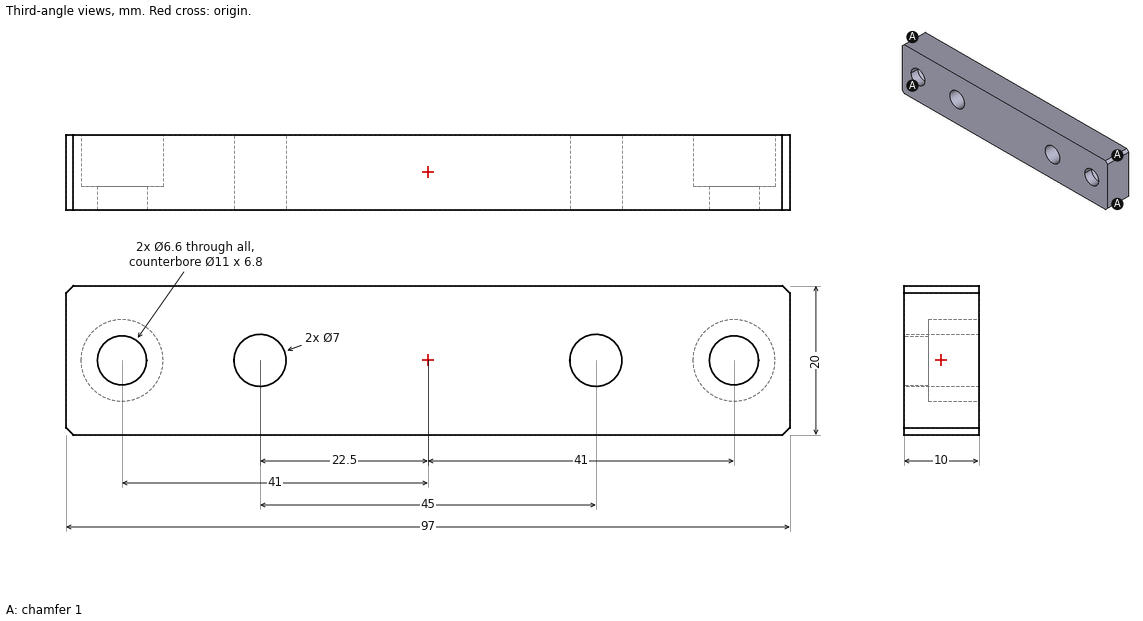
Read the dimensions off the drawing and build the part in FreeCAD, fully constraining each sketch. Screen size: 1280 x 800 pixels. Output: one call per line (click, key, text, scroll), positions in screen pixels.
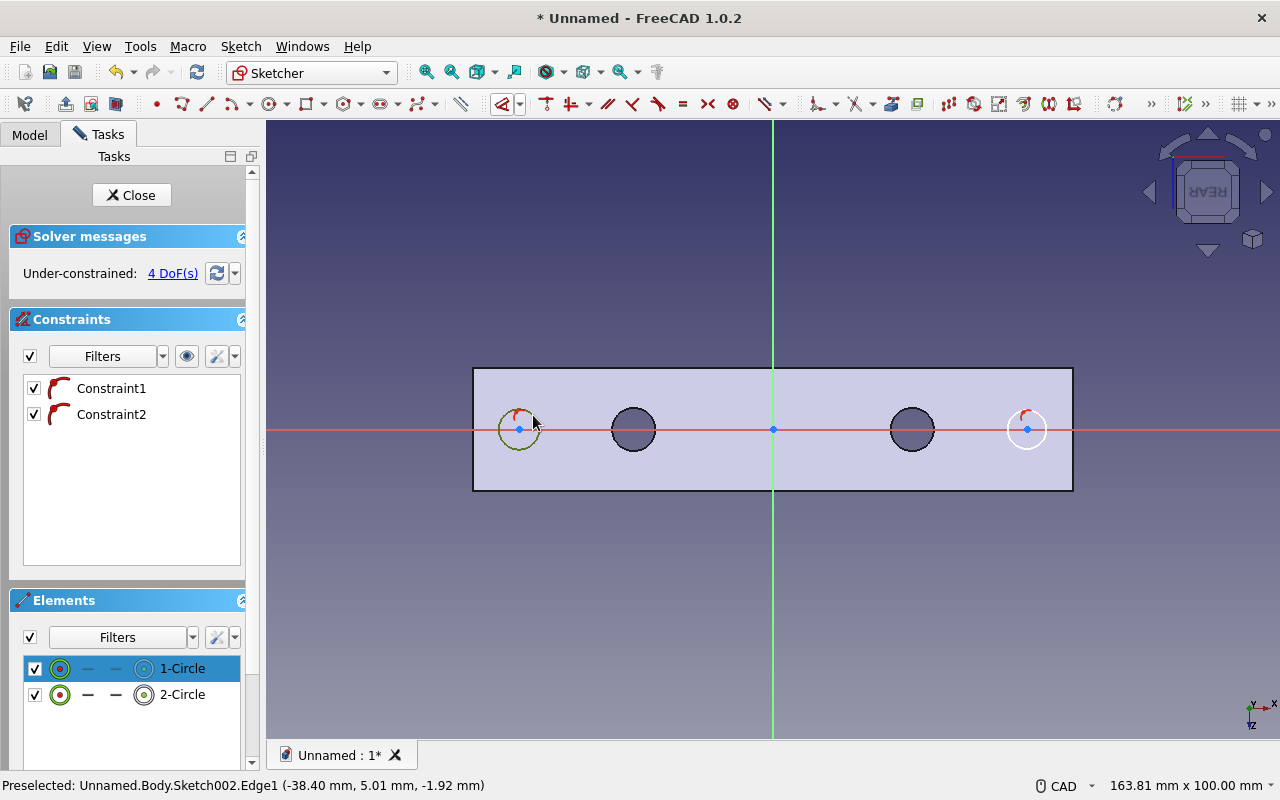
click(1041, 416)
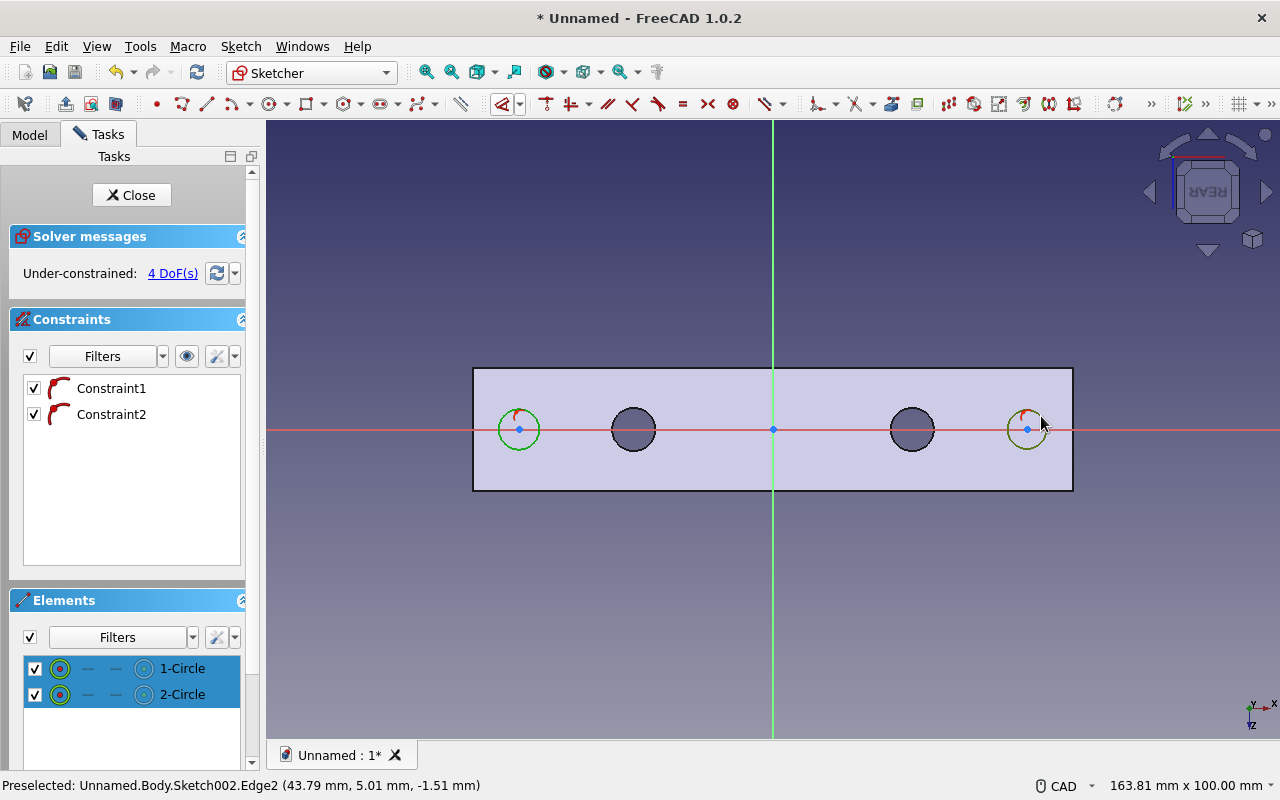
click(683, 104)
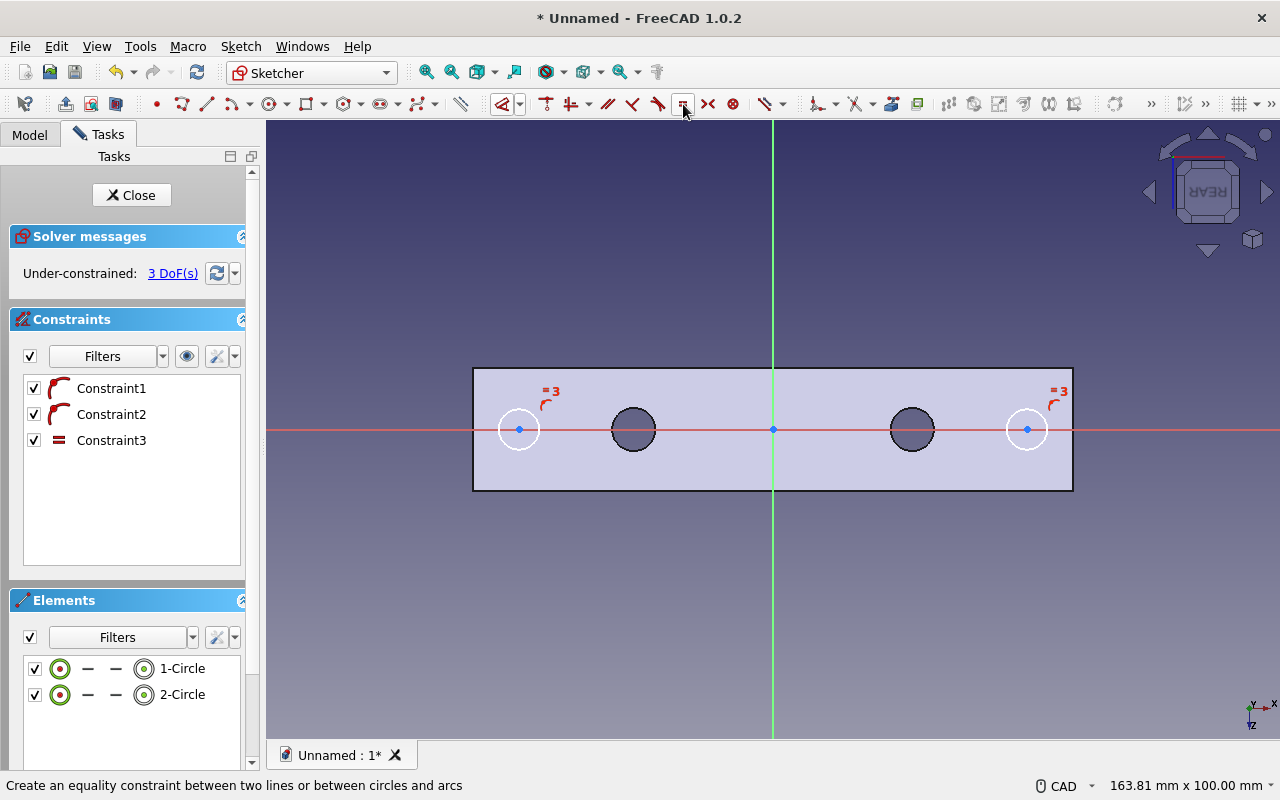
click(533, 415)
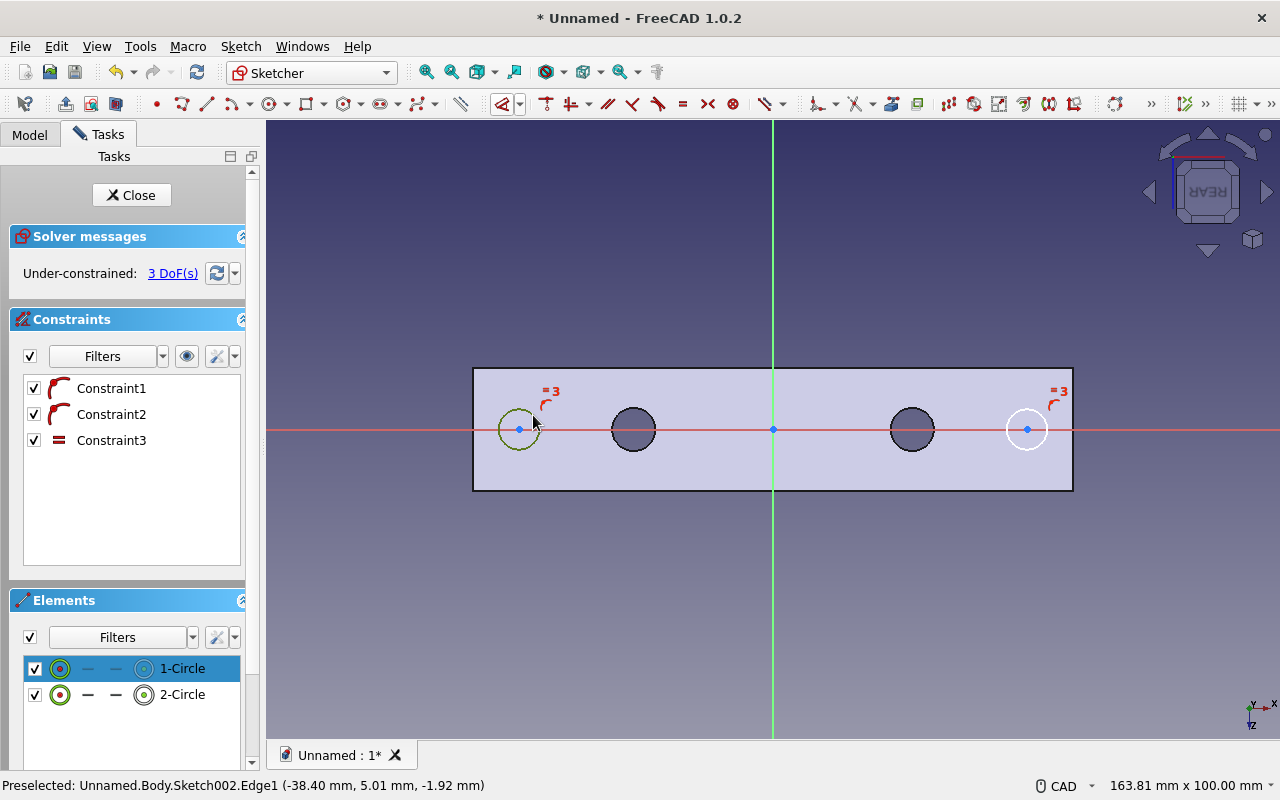
click(520, 104)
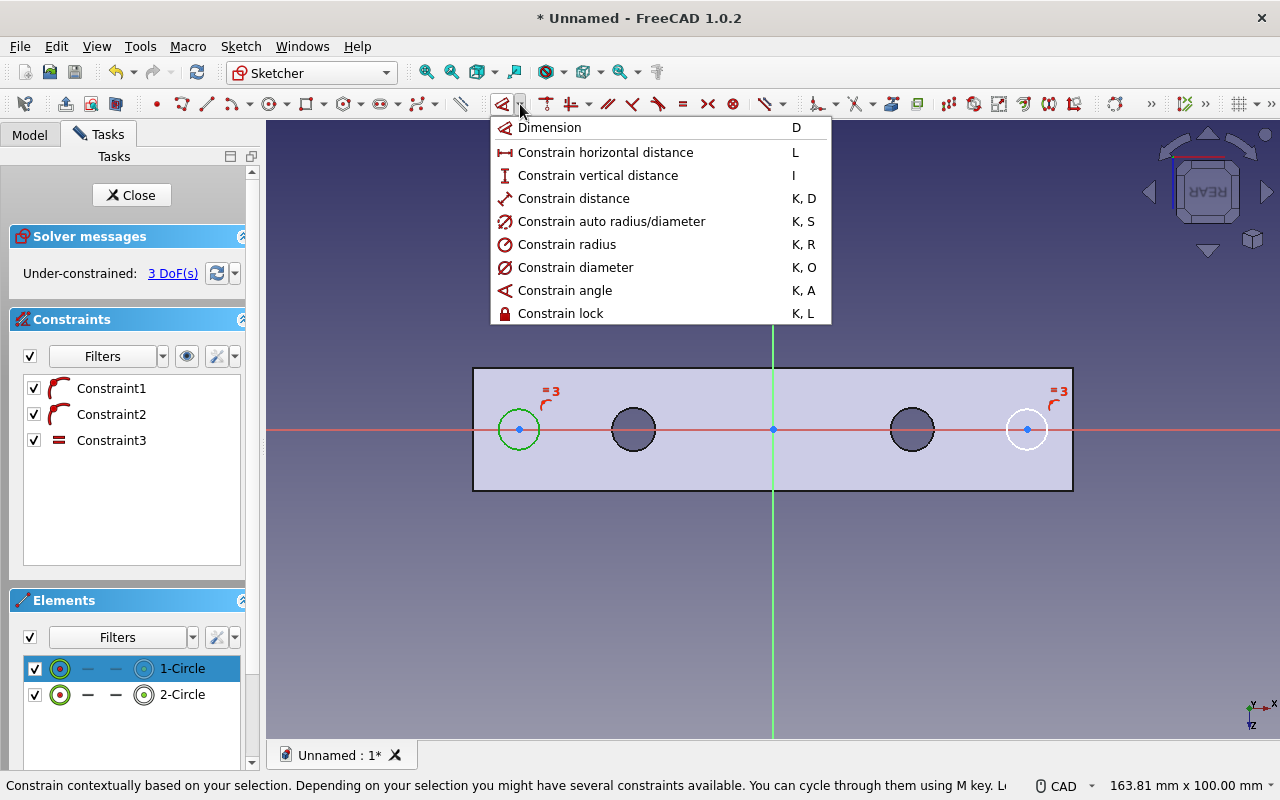
click(661, 268)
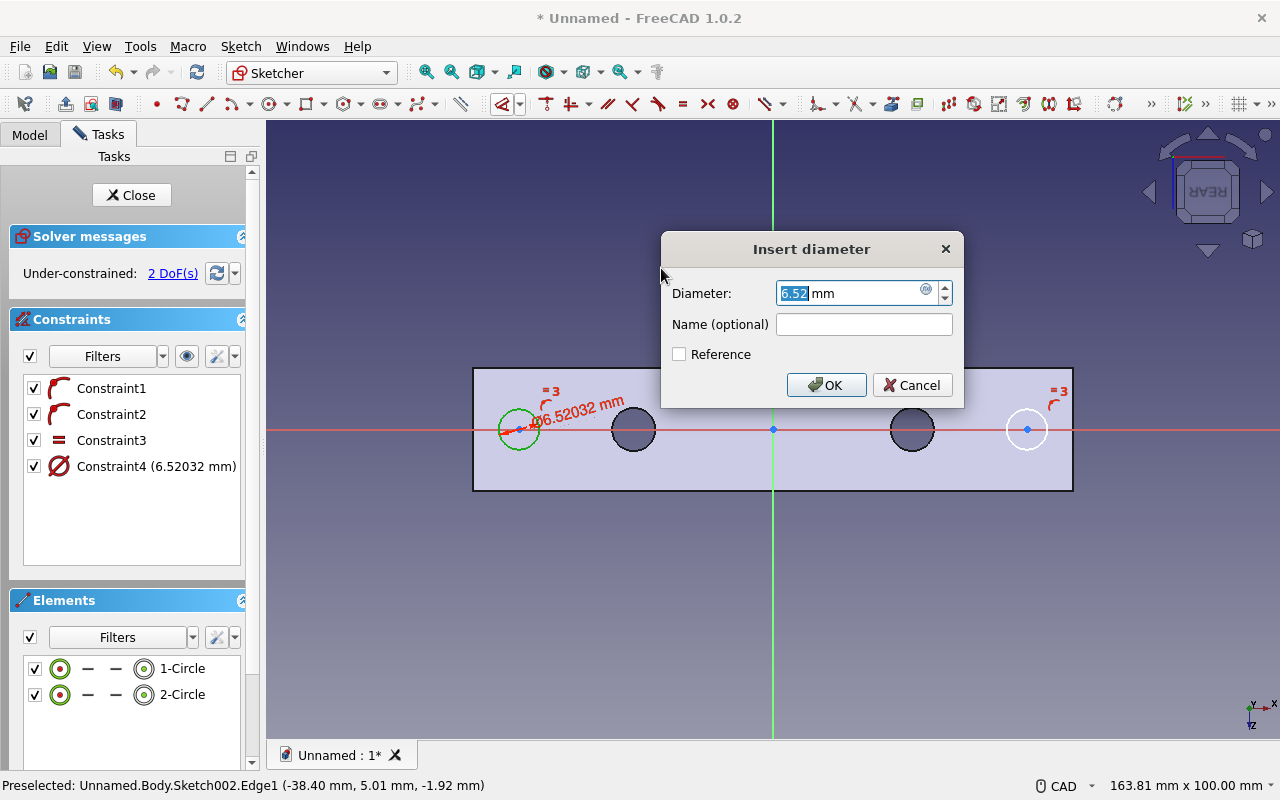
text(6.6)
key(Return)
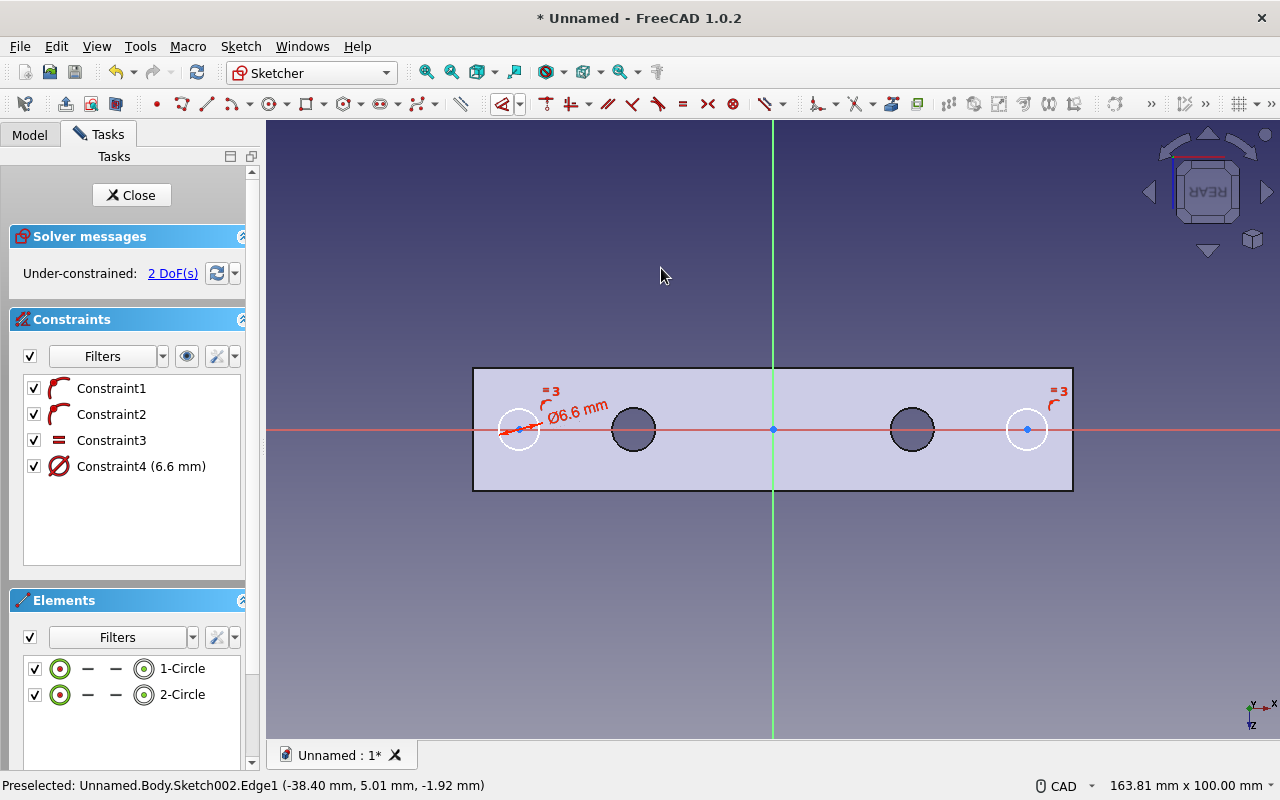
click(519, 429)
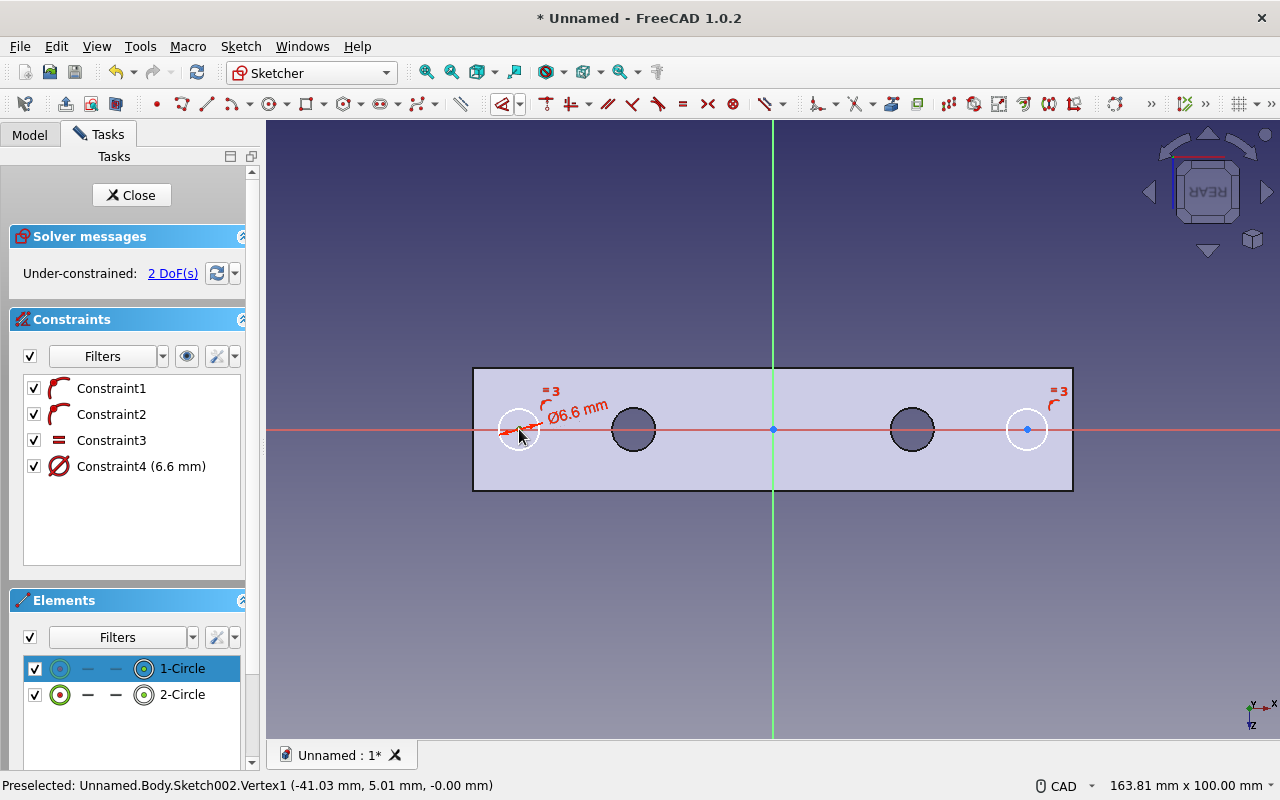
key(l)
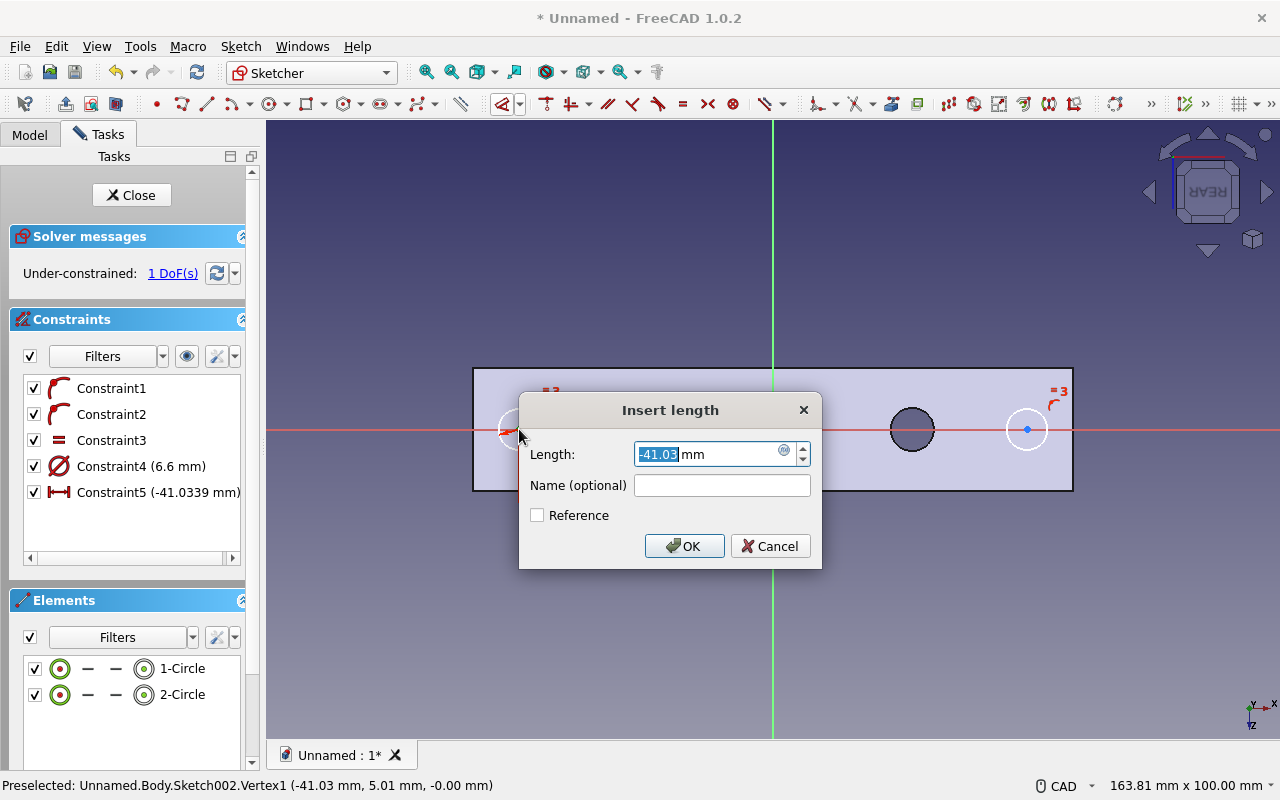
text(-41)
key(Return)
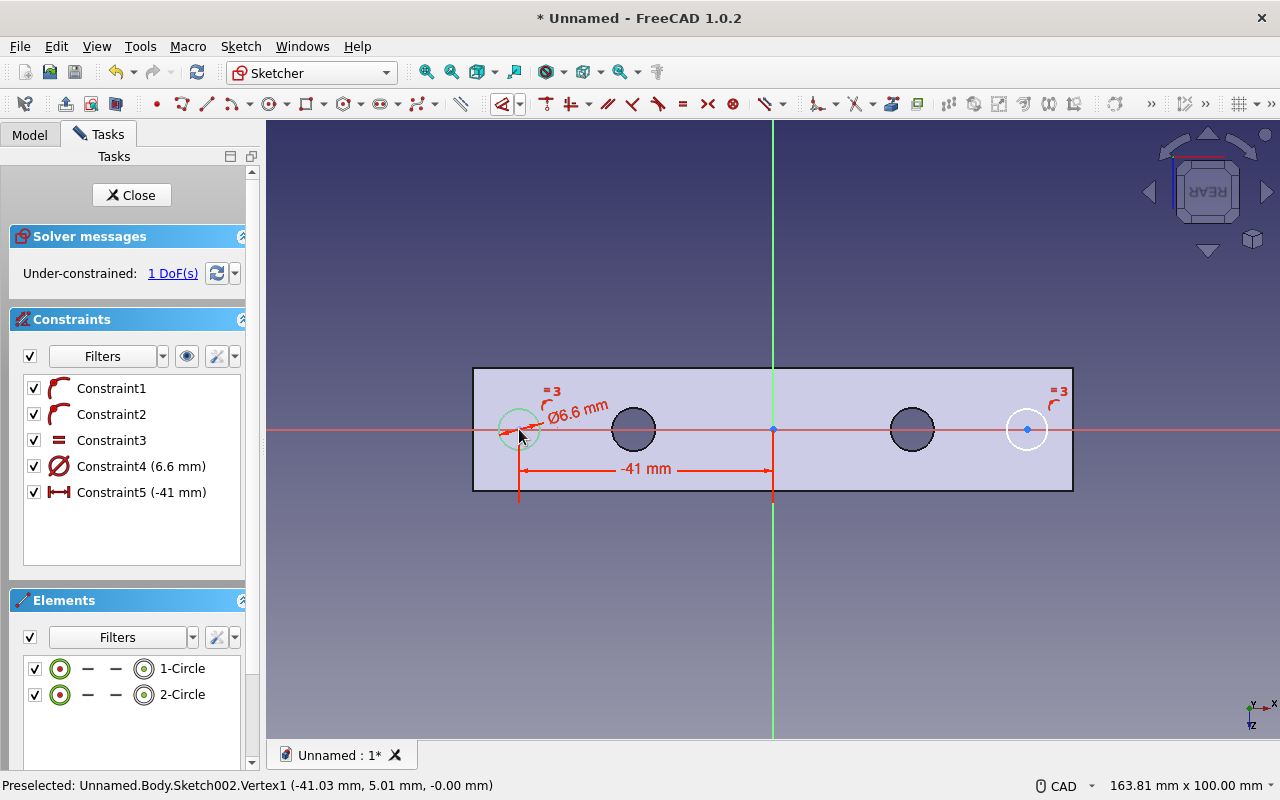
click(1027, 429)